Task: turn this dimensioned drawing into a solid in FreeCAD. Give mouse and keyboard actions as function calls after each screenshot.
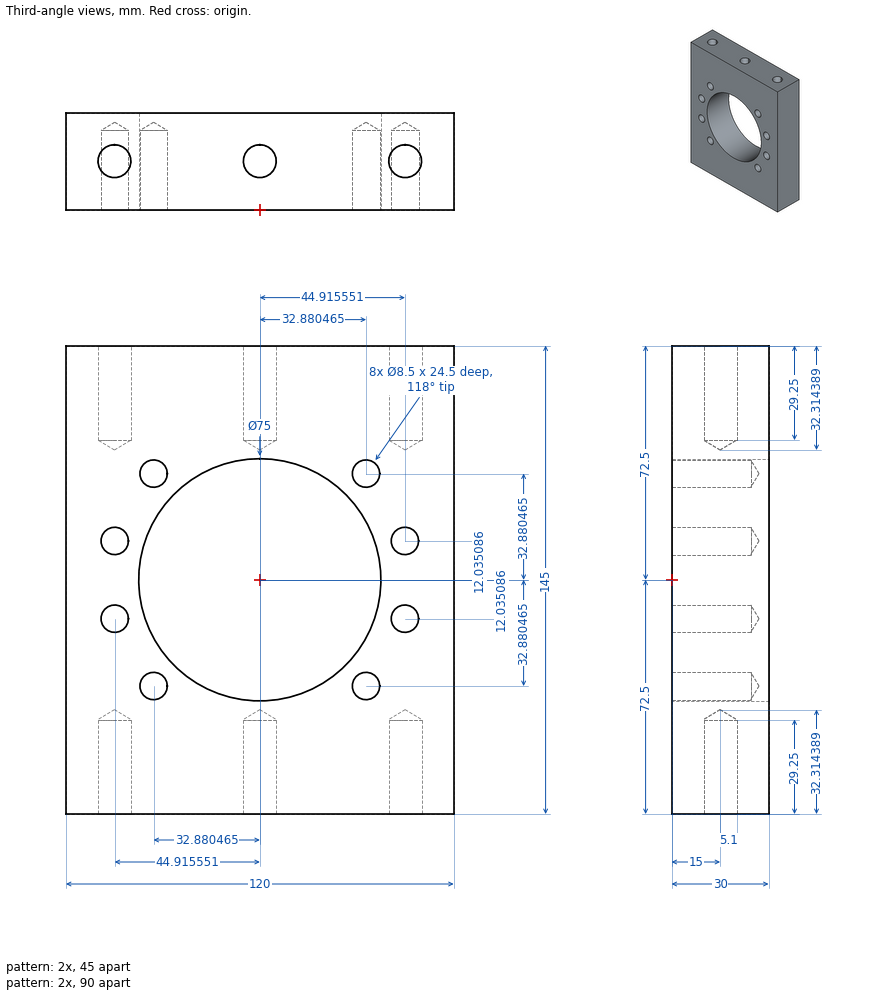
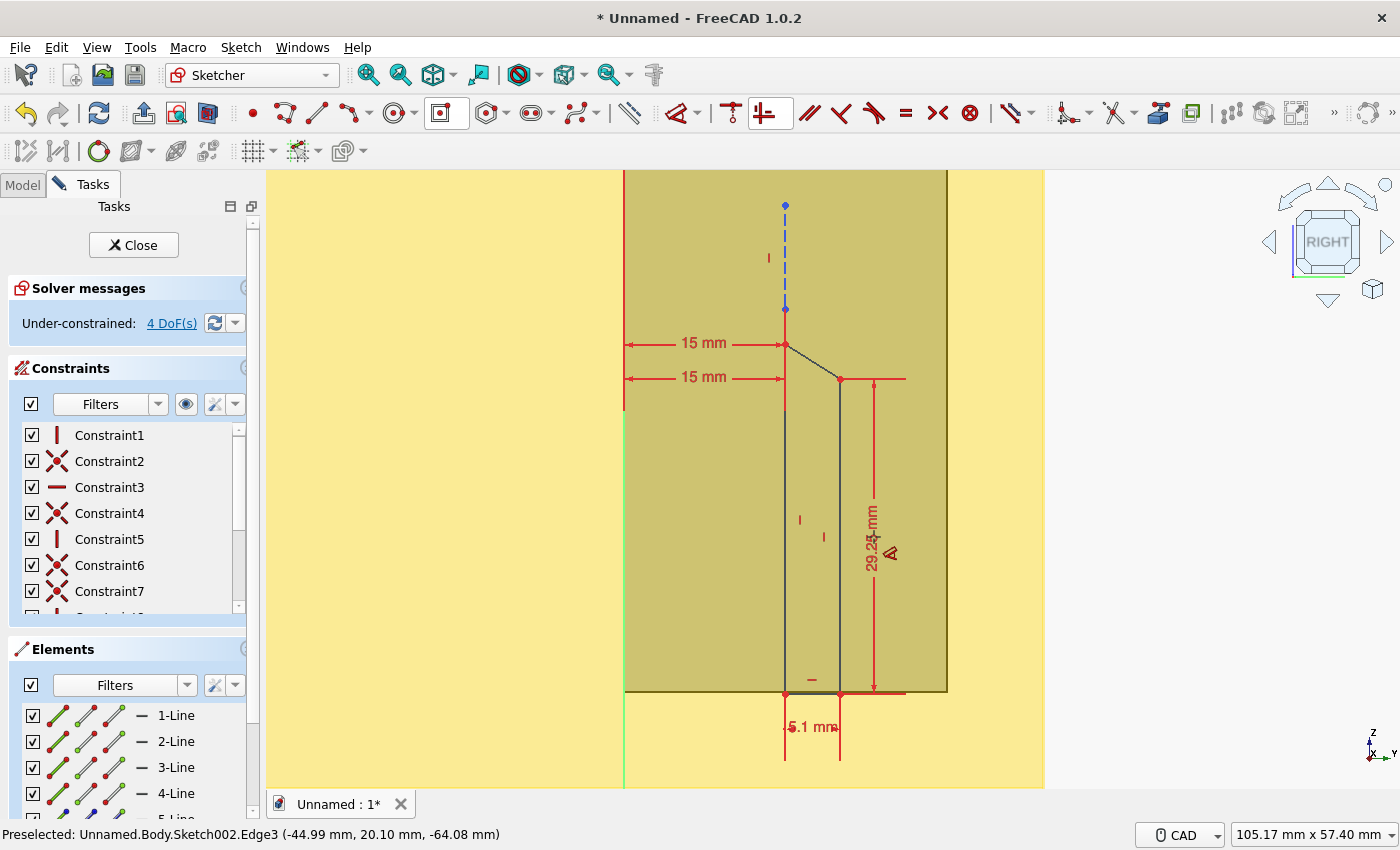
click(785, 694)
click(590, 446)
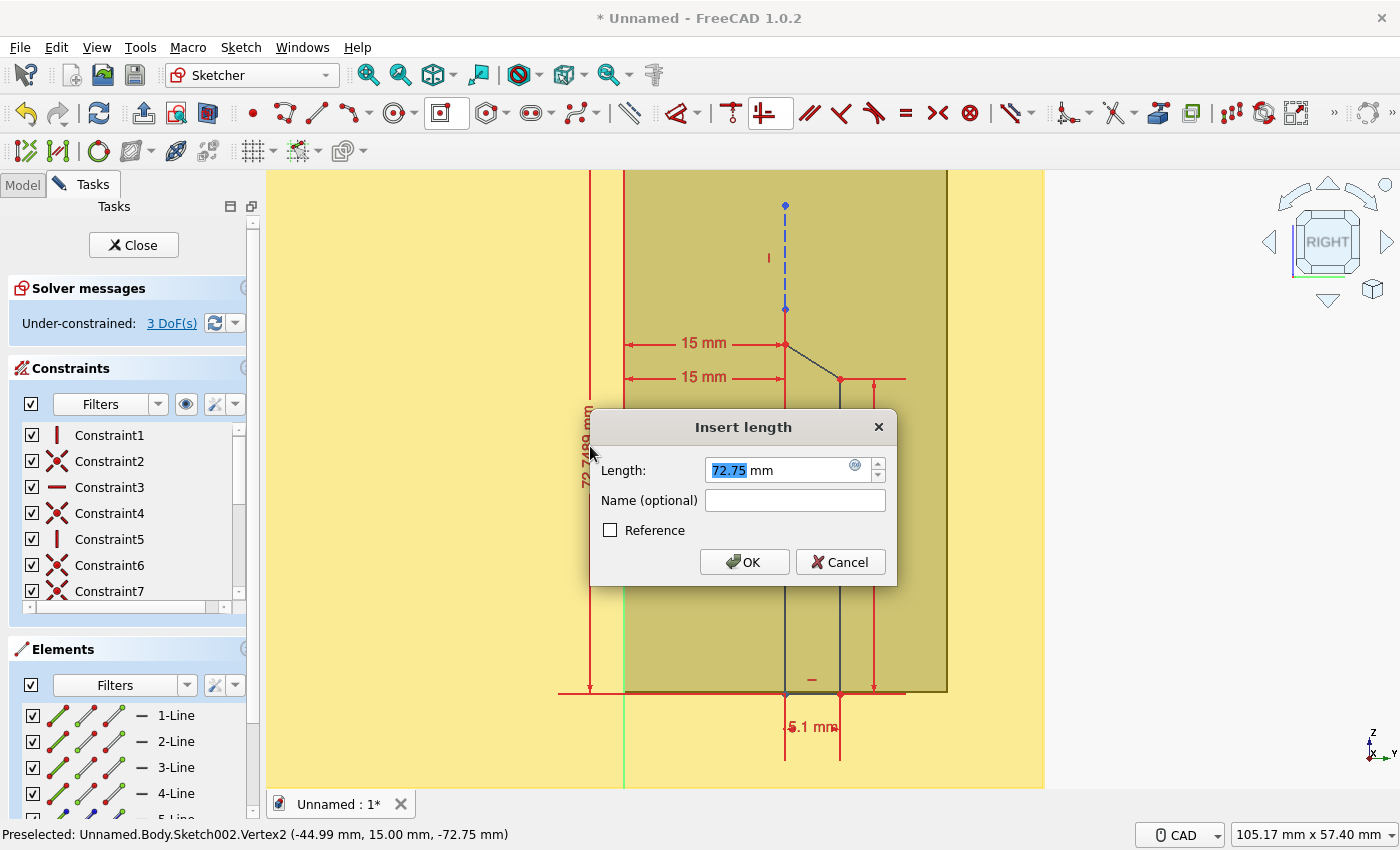
text(72.5)
key(Return)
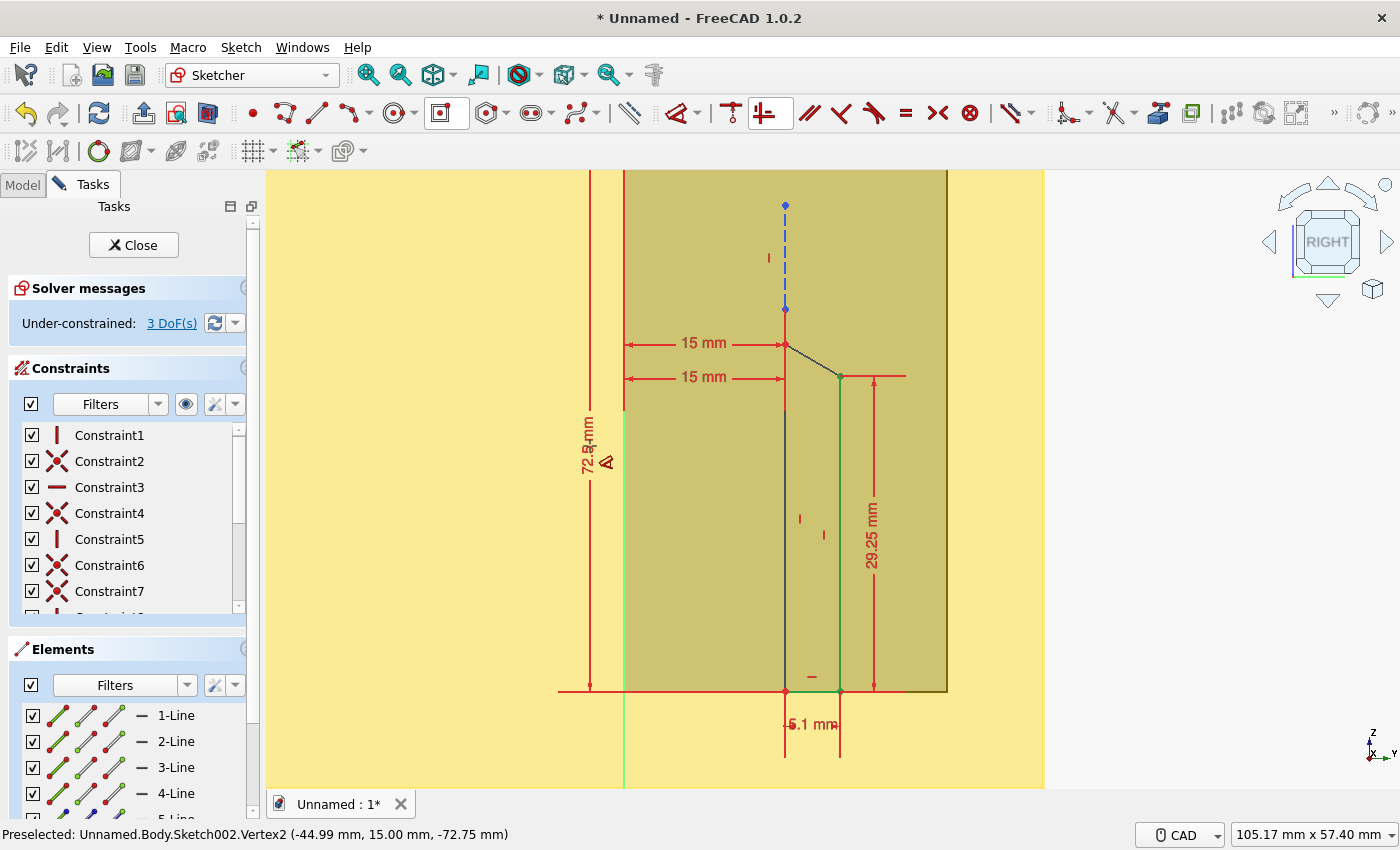
click(785, 449)
click(819, 438)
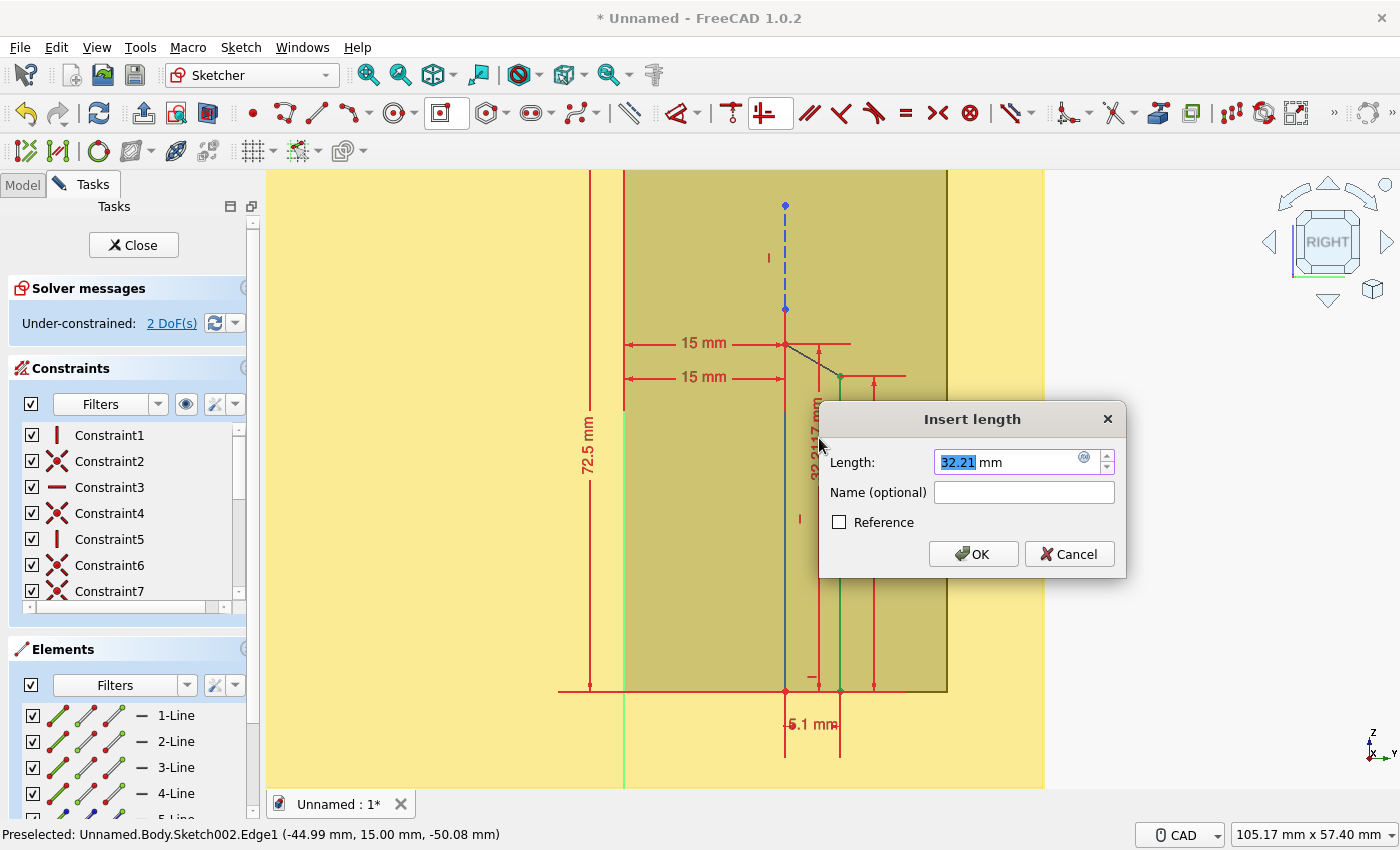
text(32.314389)
key(Return)
key(Escape)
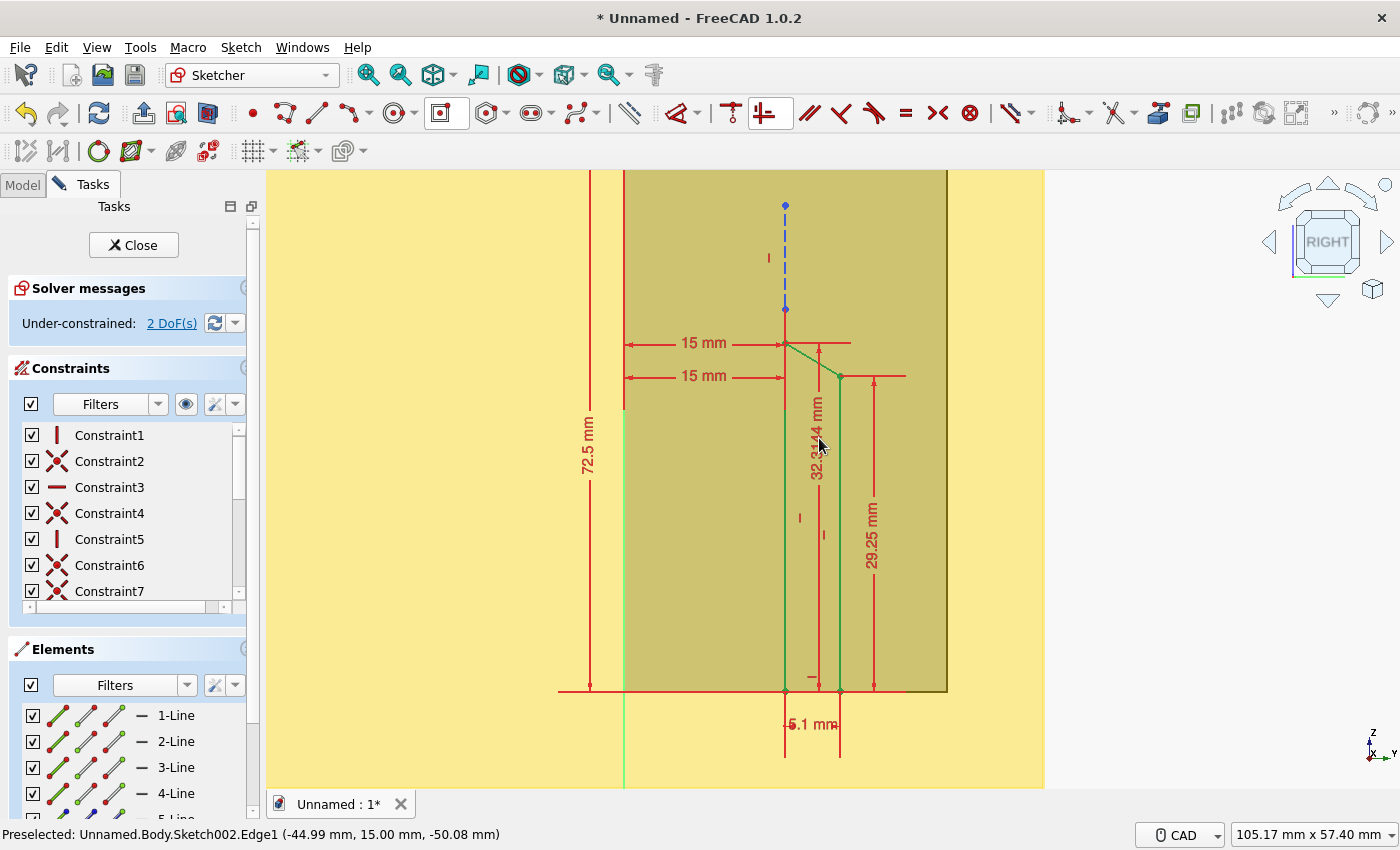
click(134, 245)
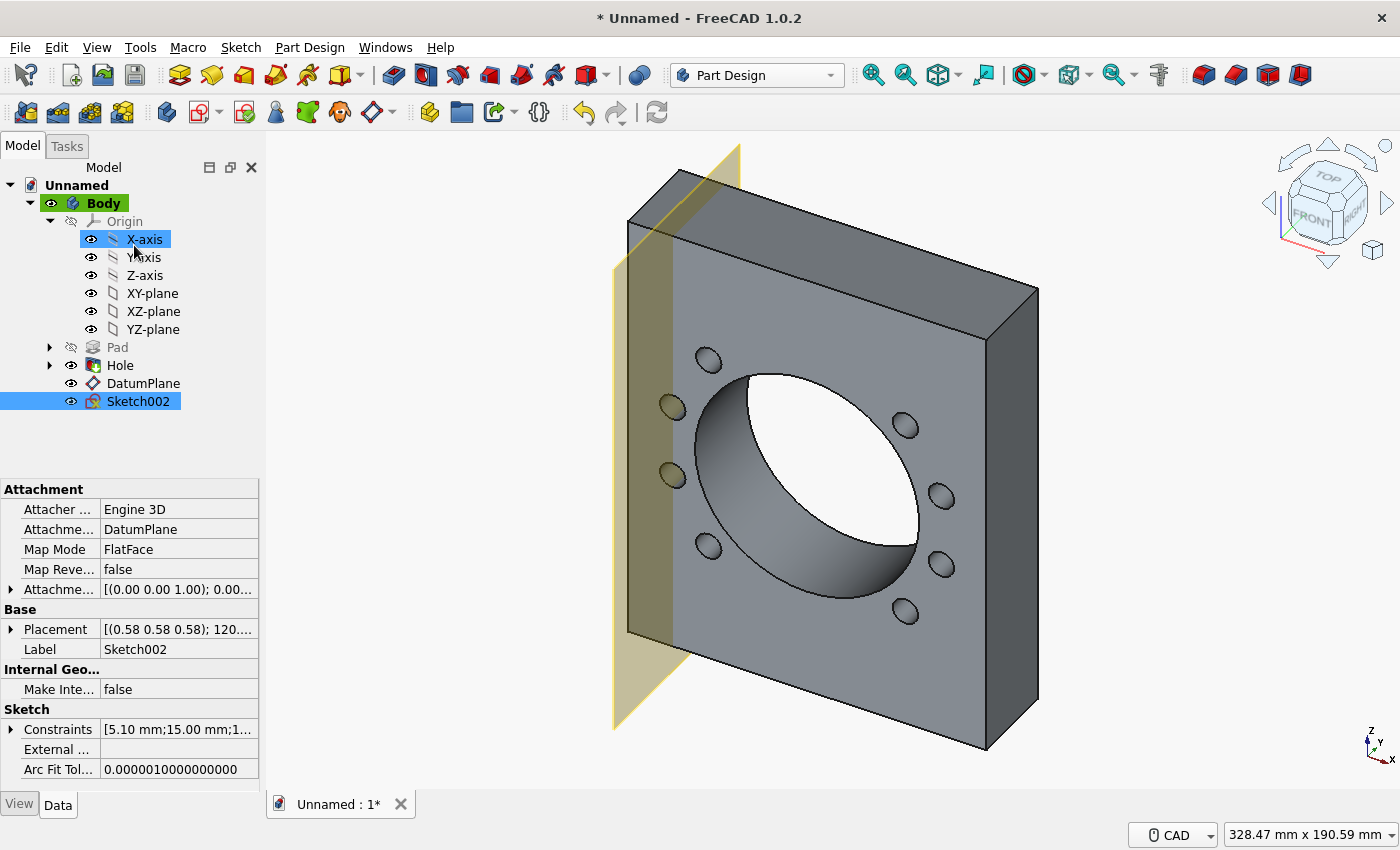
click(458, 76)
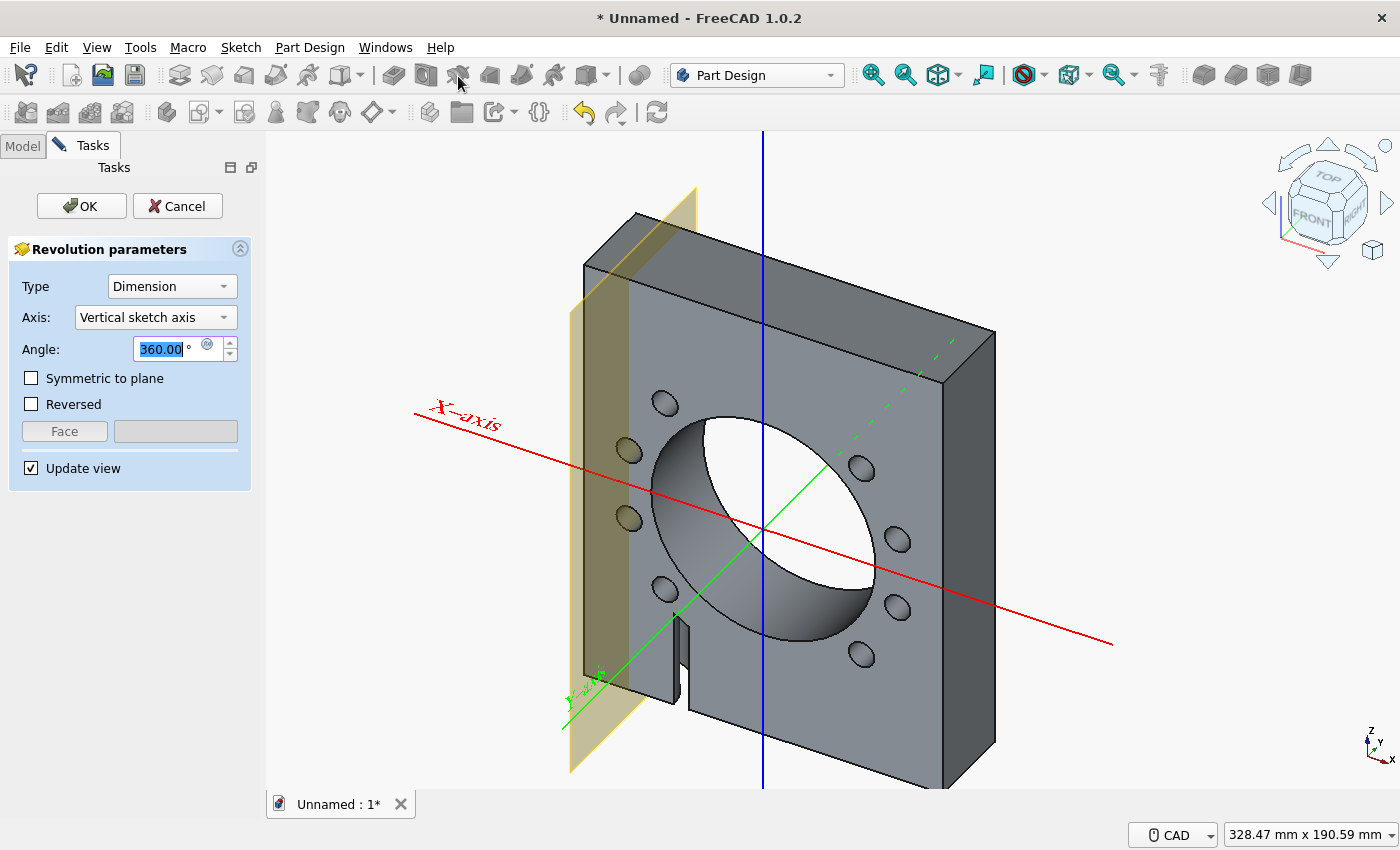
click(156, 318)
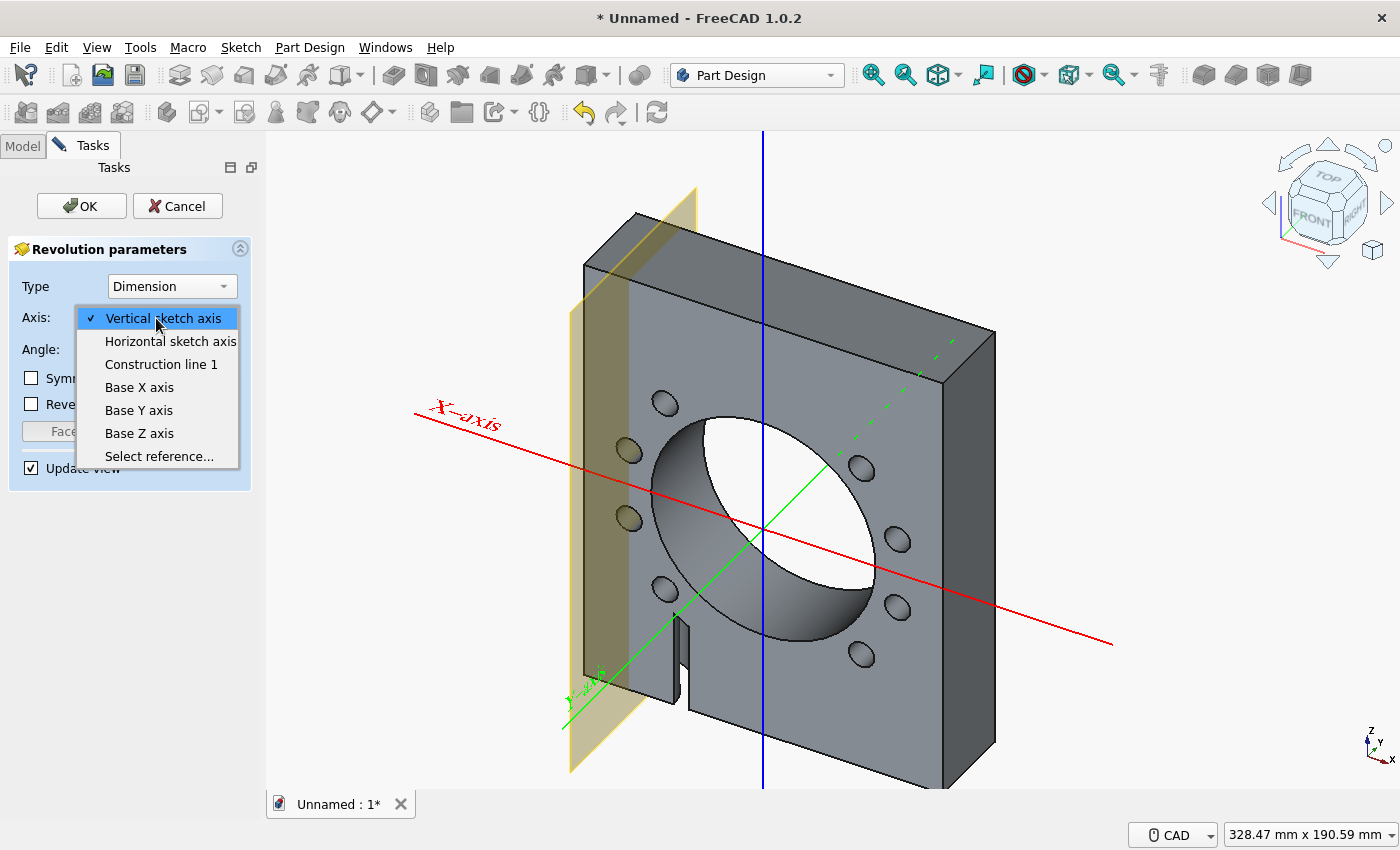
click(156, 364)